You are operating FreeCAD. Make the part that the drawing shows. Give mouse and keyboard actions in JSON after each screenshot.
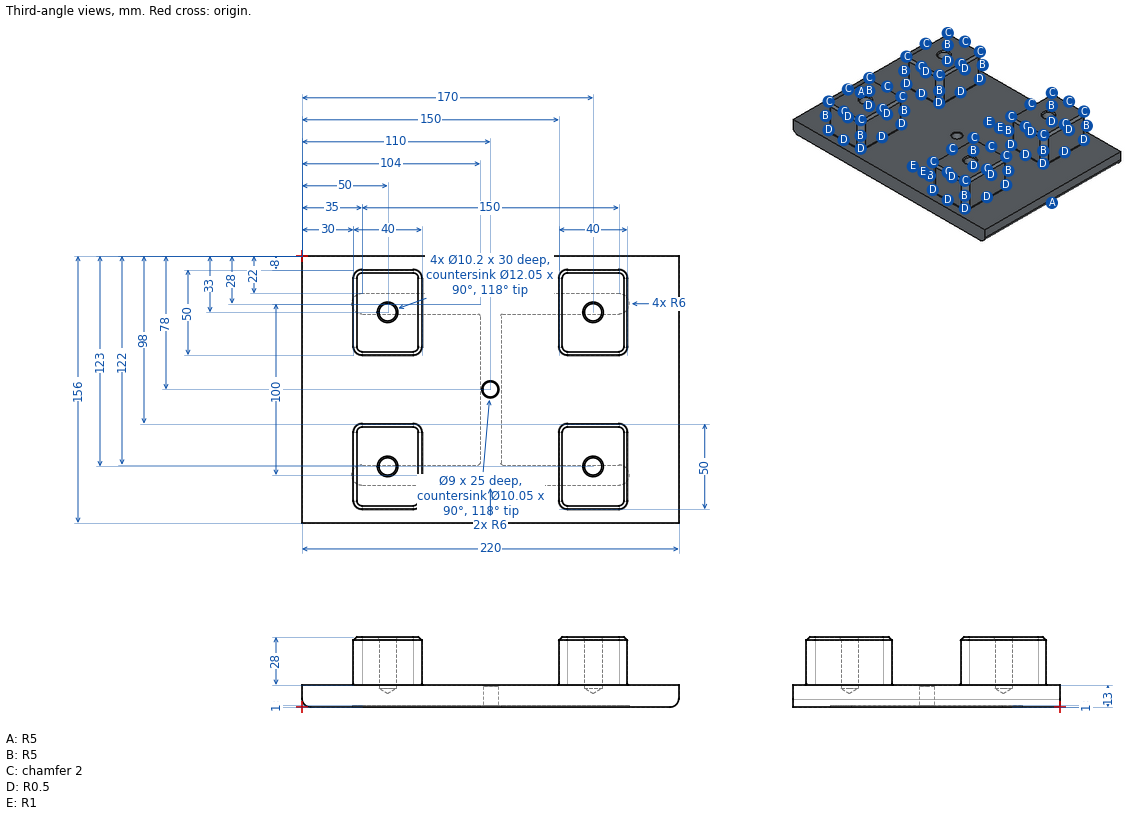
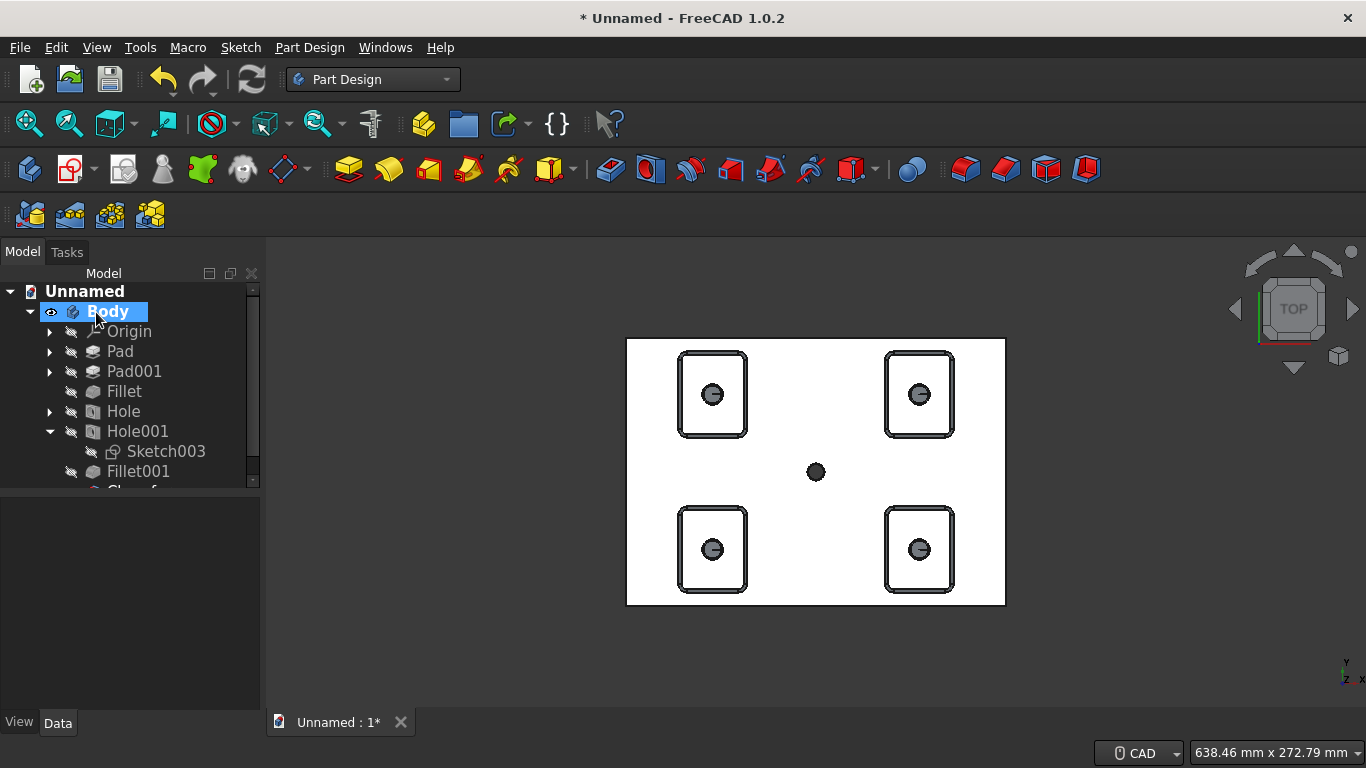
{"action": "key", "text": "5"}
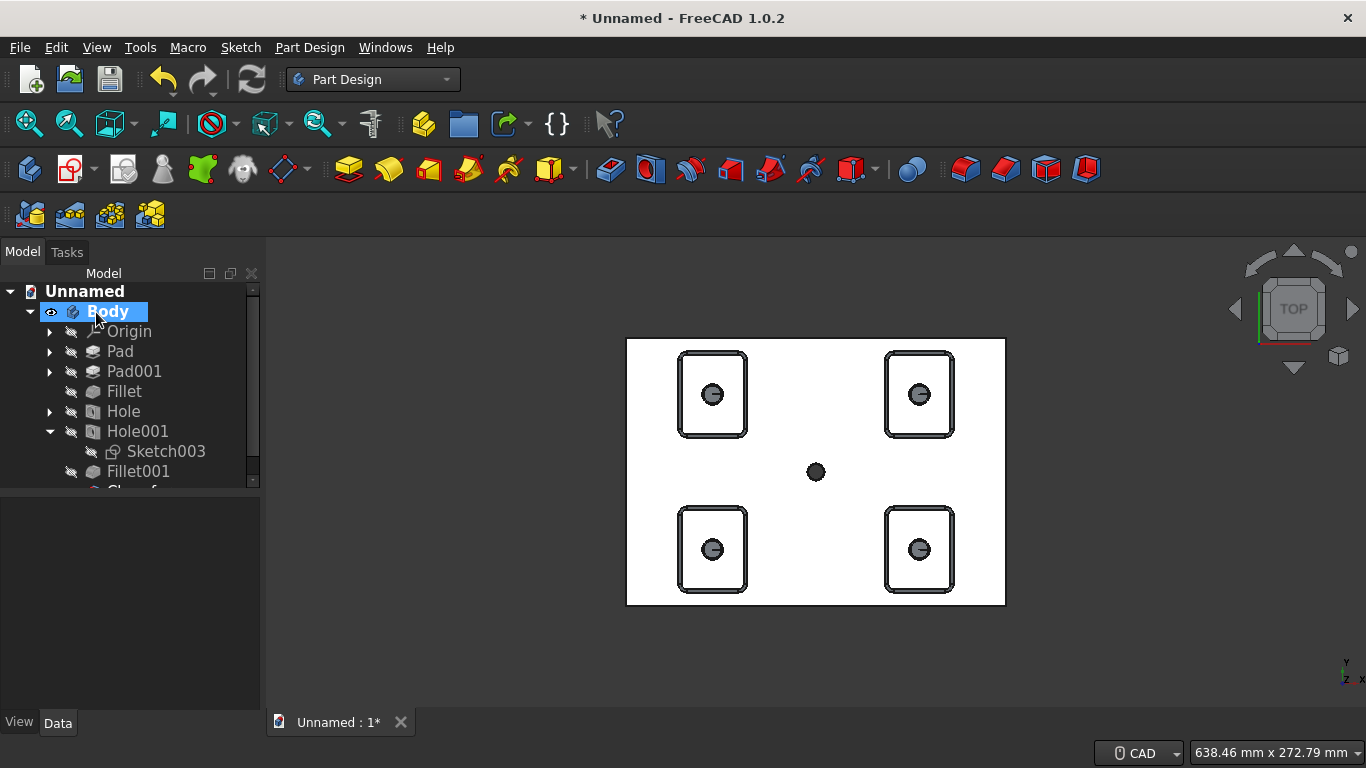
{"action": "left_click", "coordinate": [919, 509]}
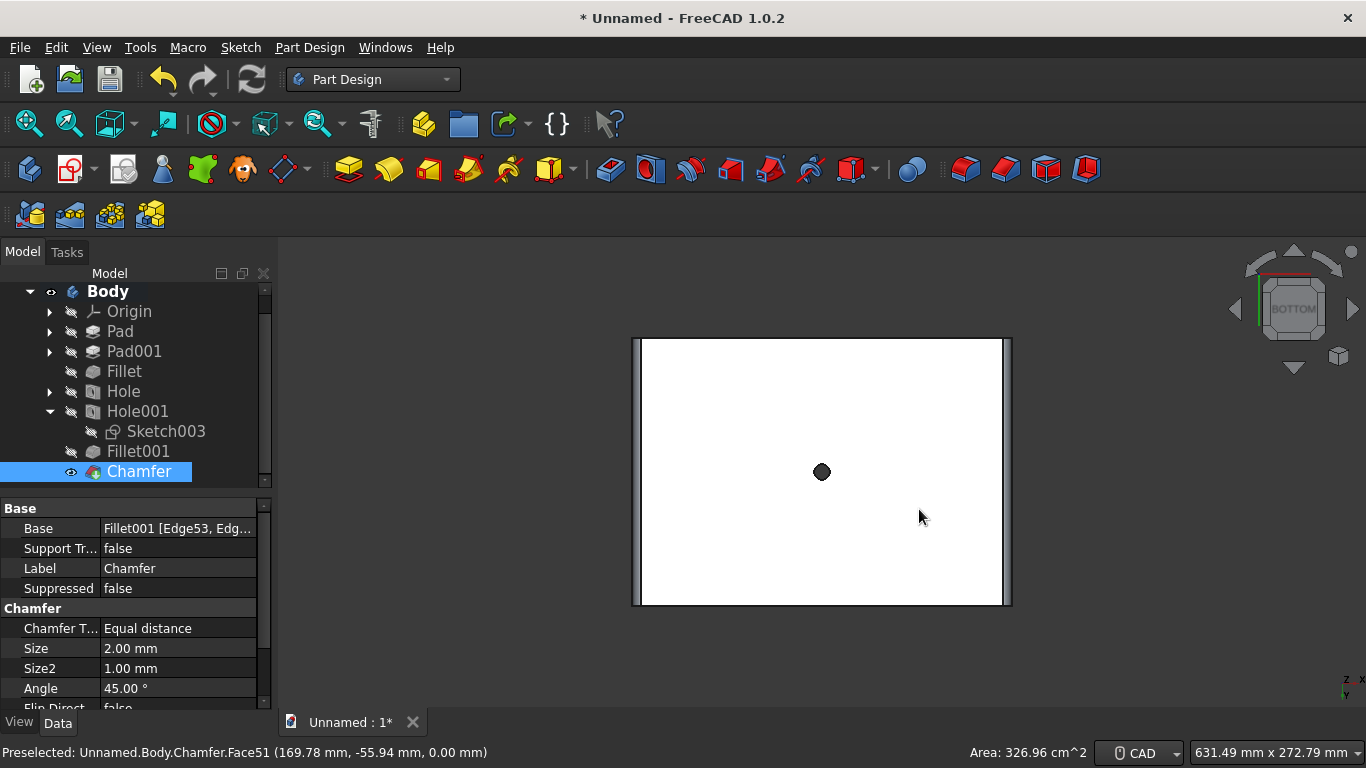
{"action": "left_click", "coordinate": [70, 170]}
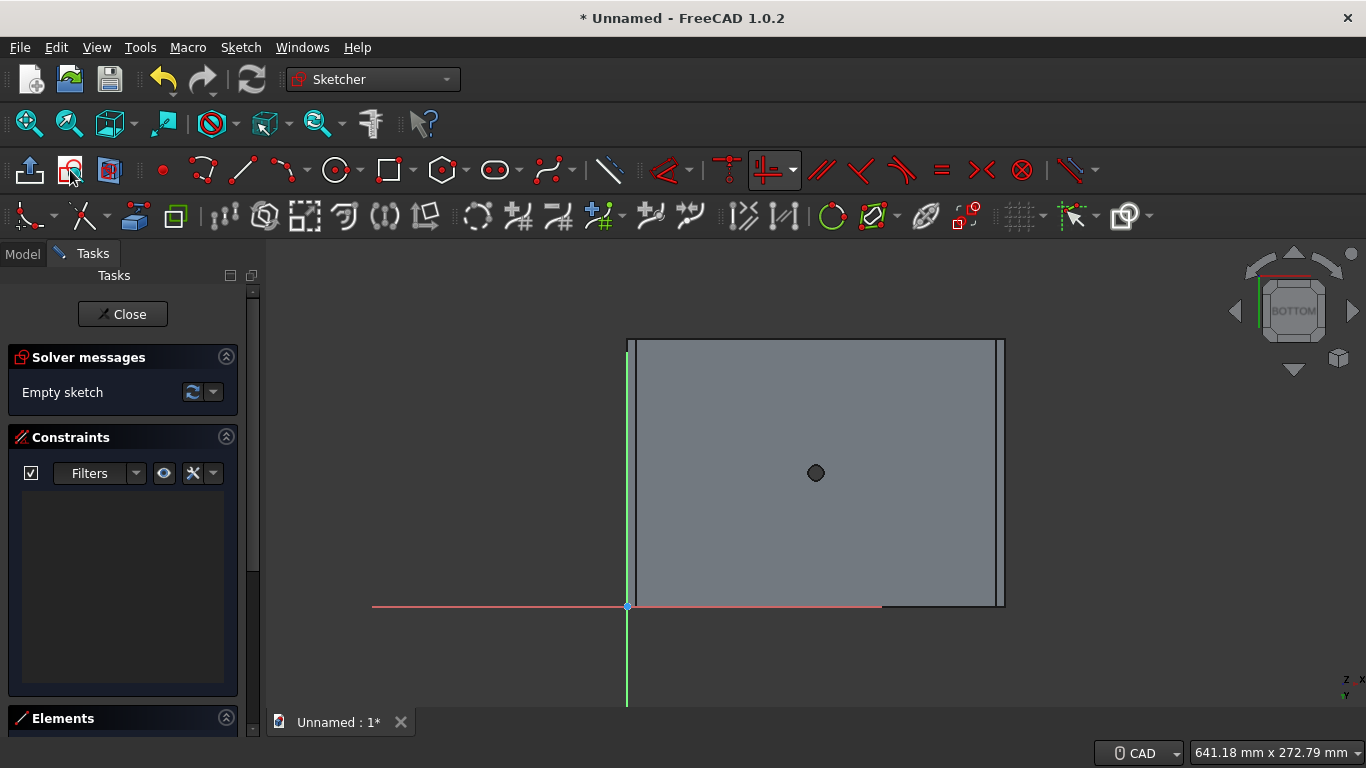
{"action": "key", "text": "g s"}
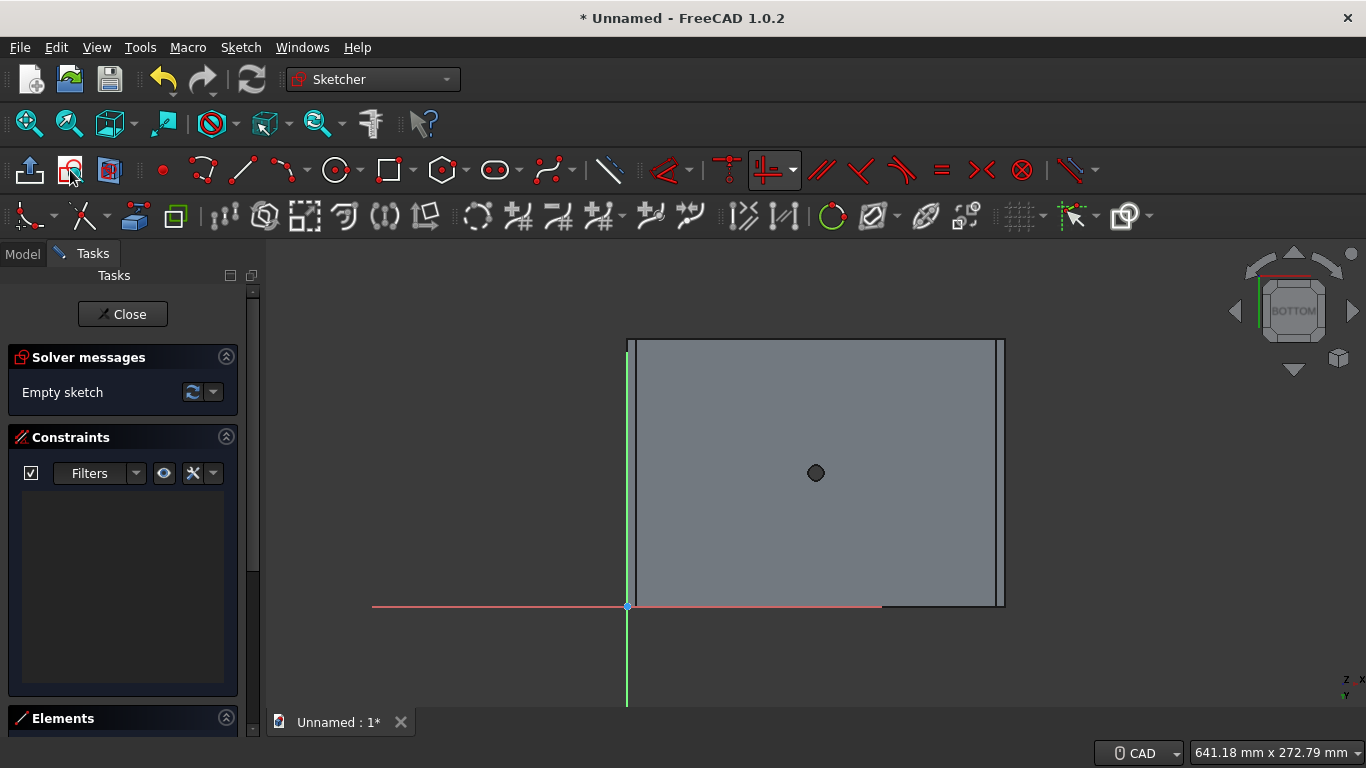
{"action": "scroll", "coordinate": [816, 559], "scroll_direction": "up", "scroll_amount": 4}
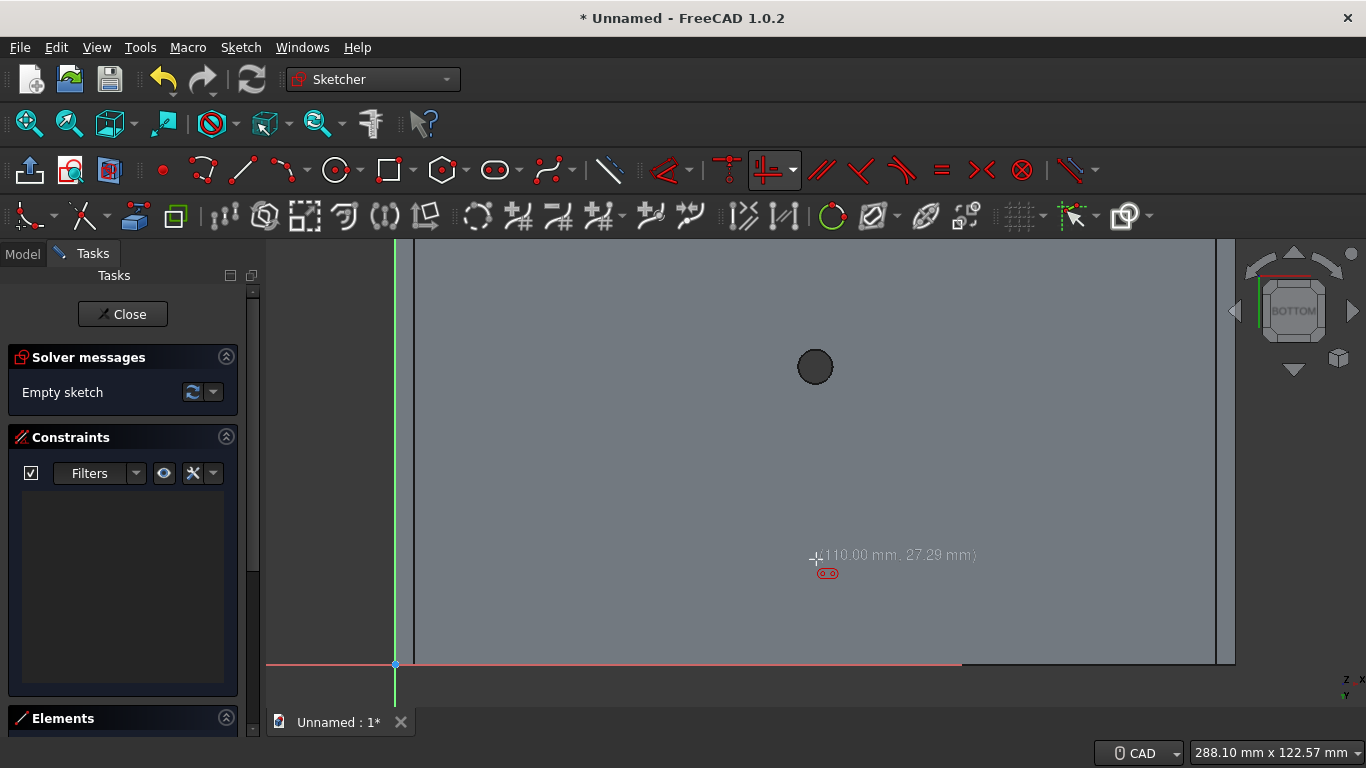
{"action": "left_click", "coordinate": [815, 558]}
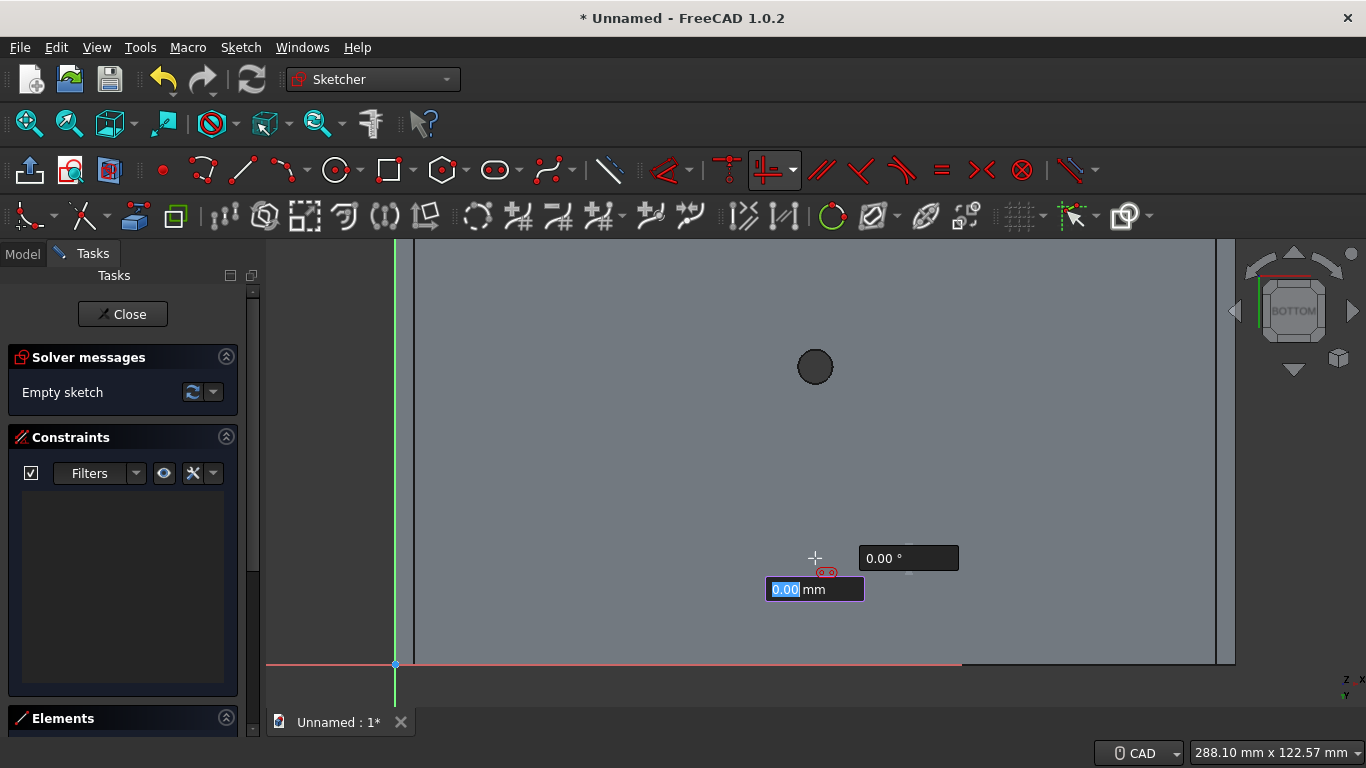
{"action": "scroll", "coordinate": [906, 551], "scroll_direction": "down", "scroll_amount": 3}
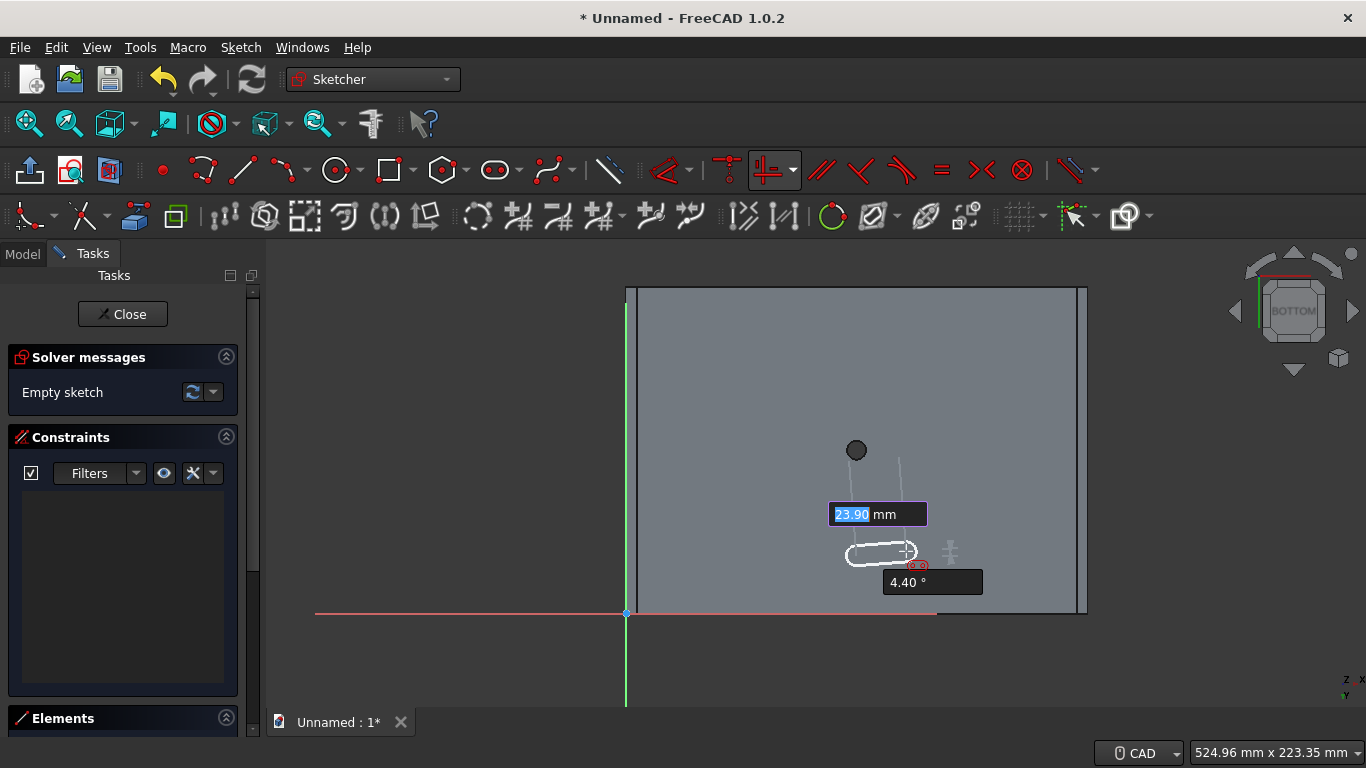
{"action": "left_click", "coordinate": [856, 345]}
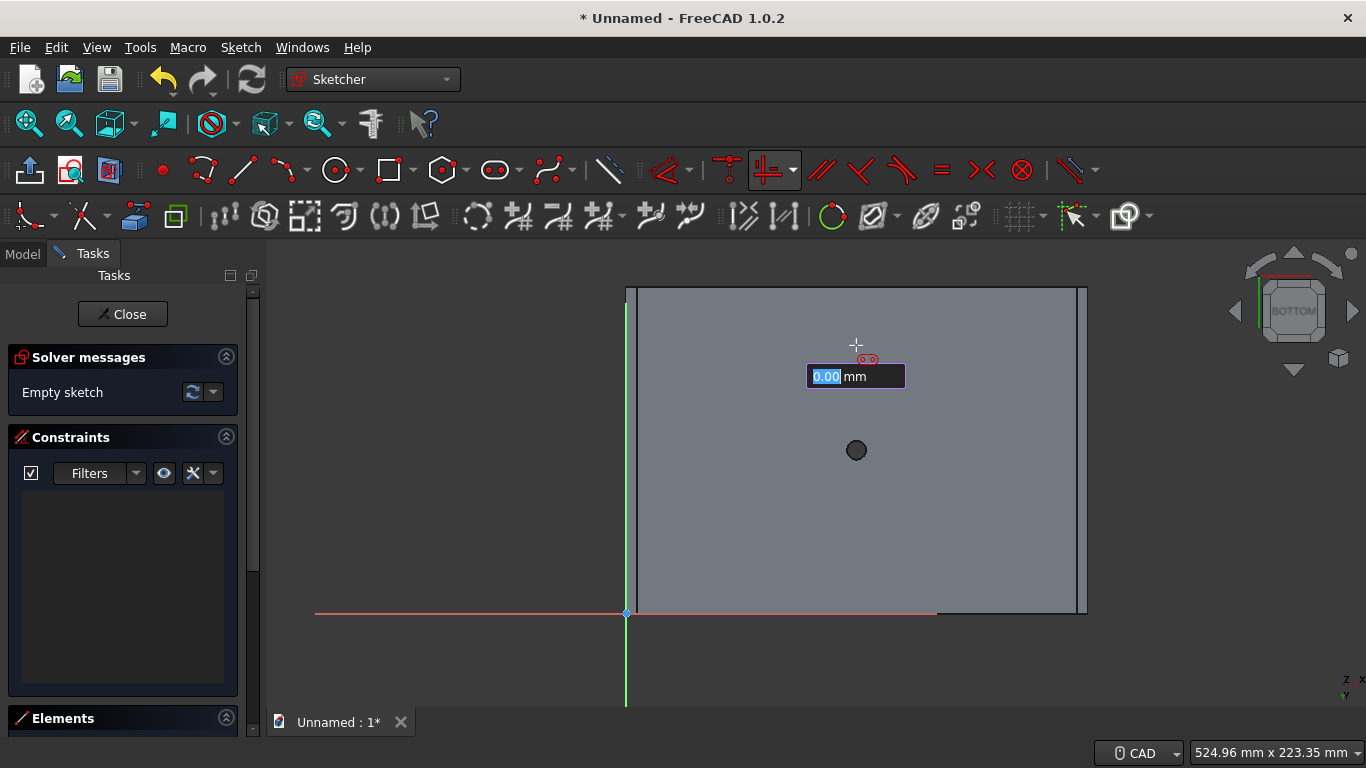
{"action": "scroll", "coordinate": [869, 450], "scroll_direction": "up", "scroll_amount": 2}